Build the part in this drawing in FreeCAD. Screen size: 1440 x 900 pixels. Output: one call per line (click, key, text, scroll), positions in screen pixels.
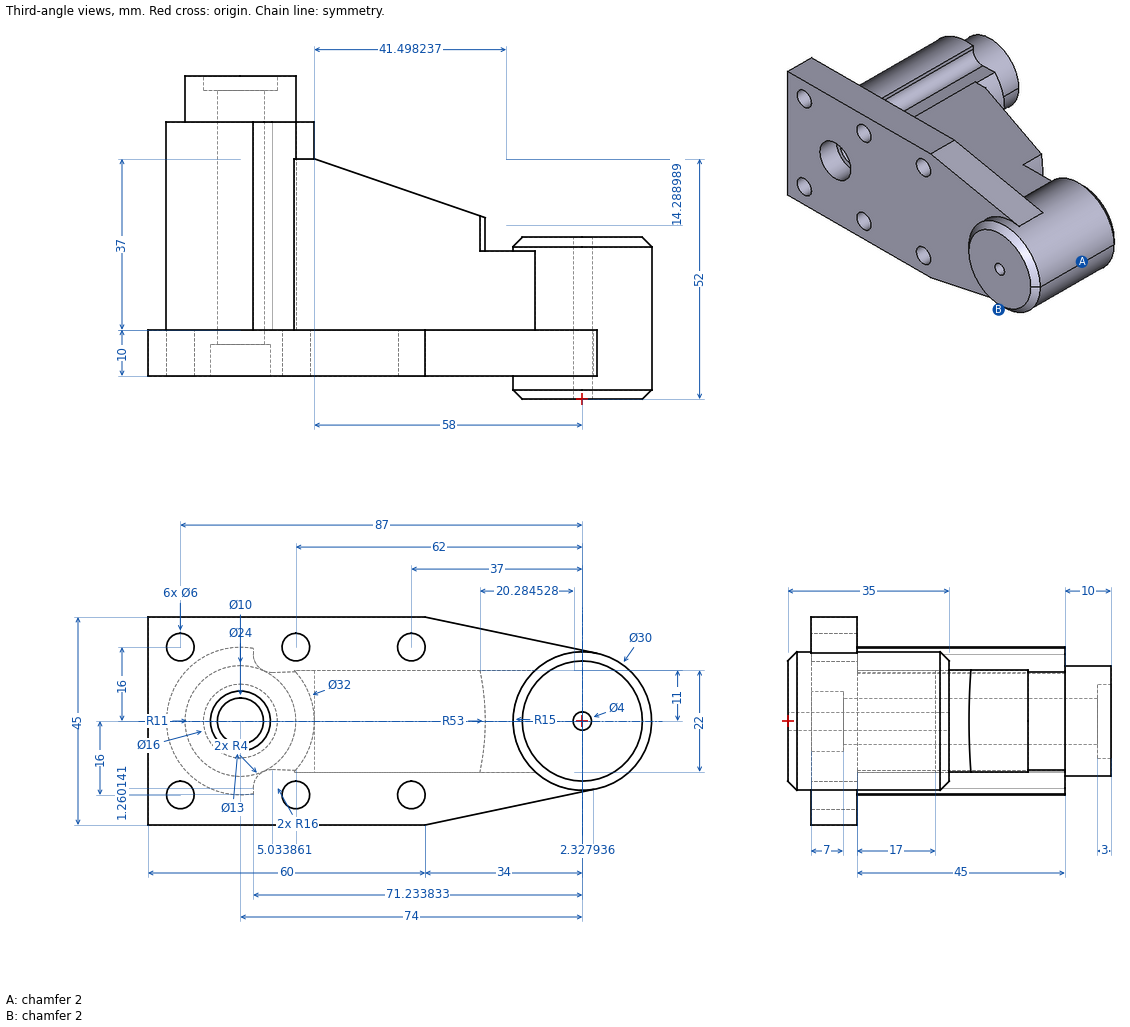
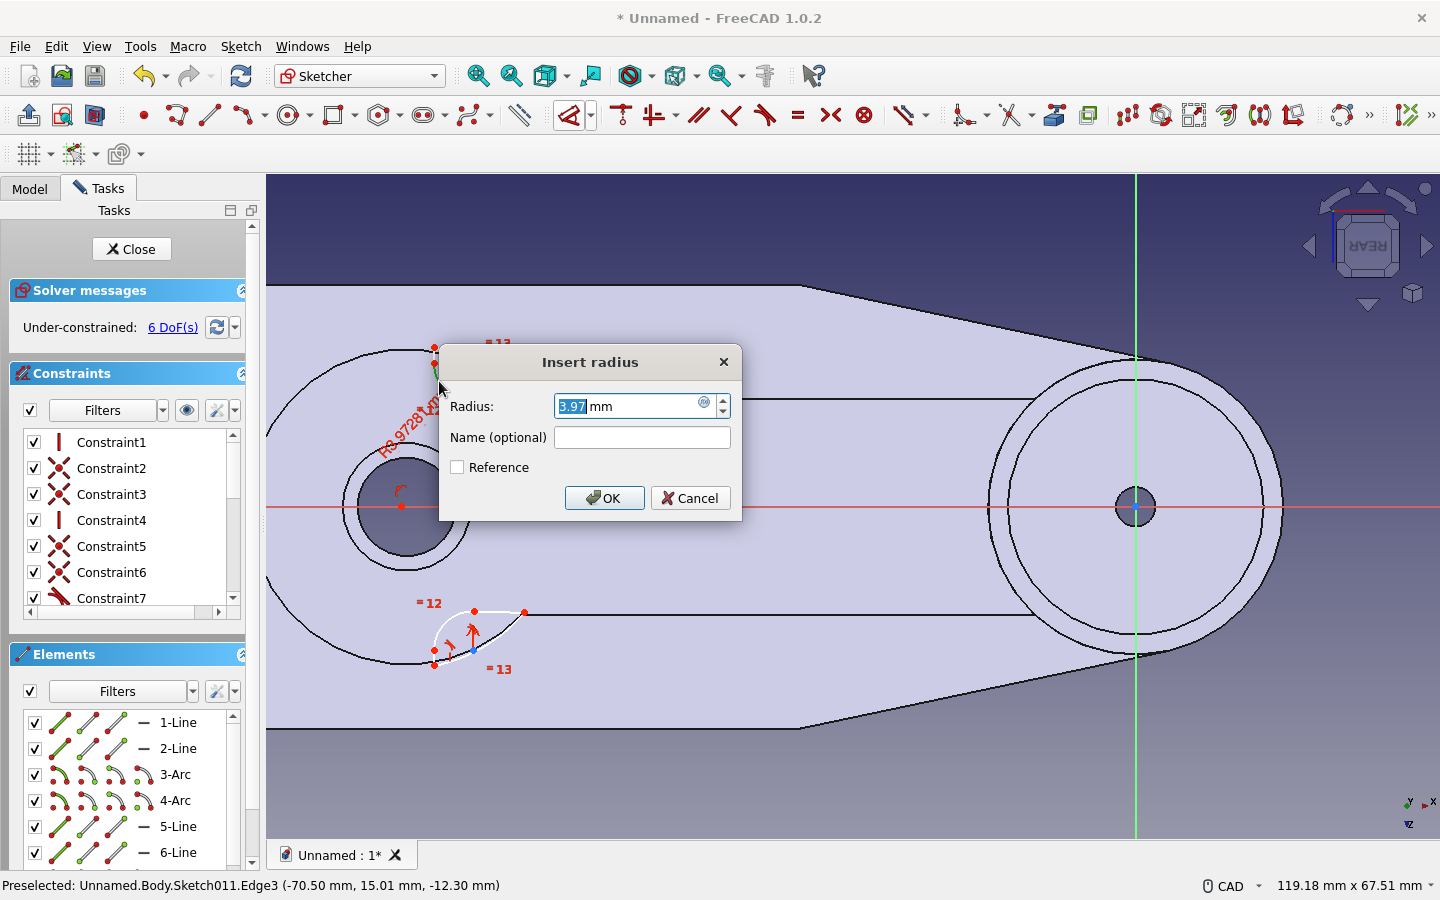
text(4)
key(Return)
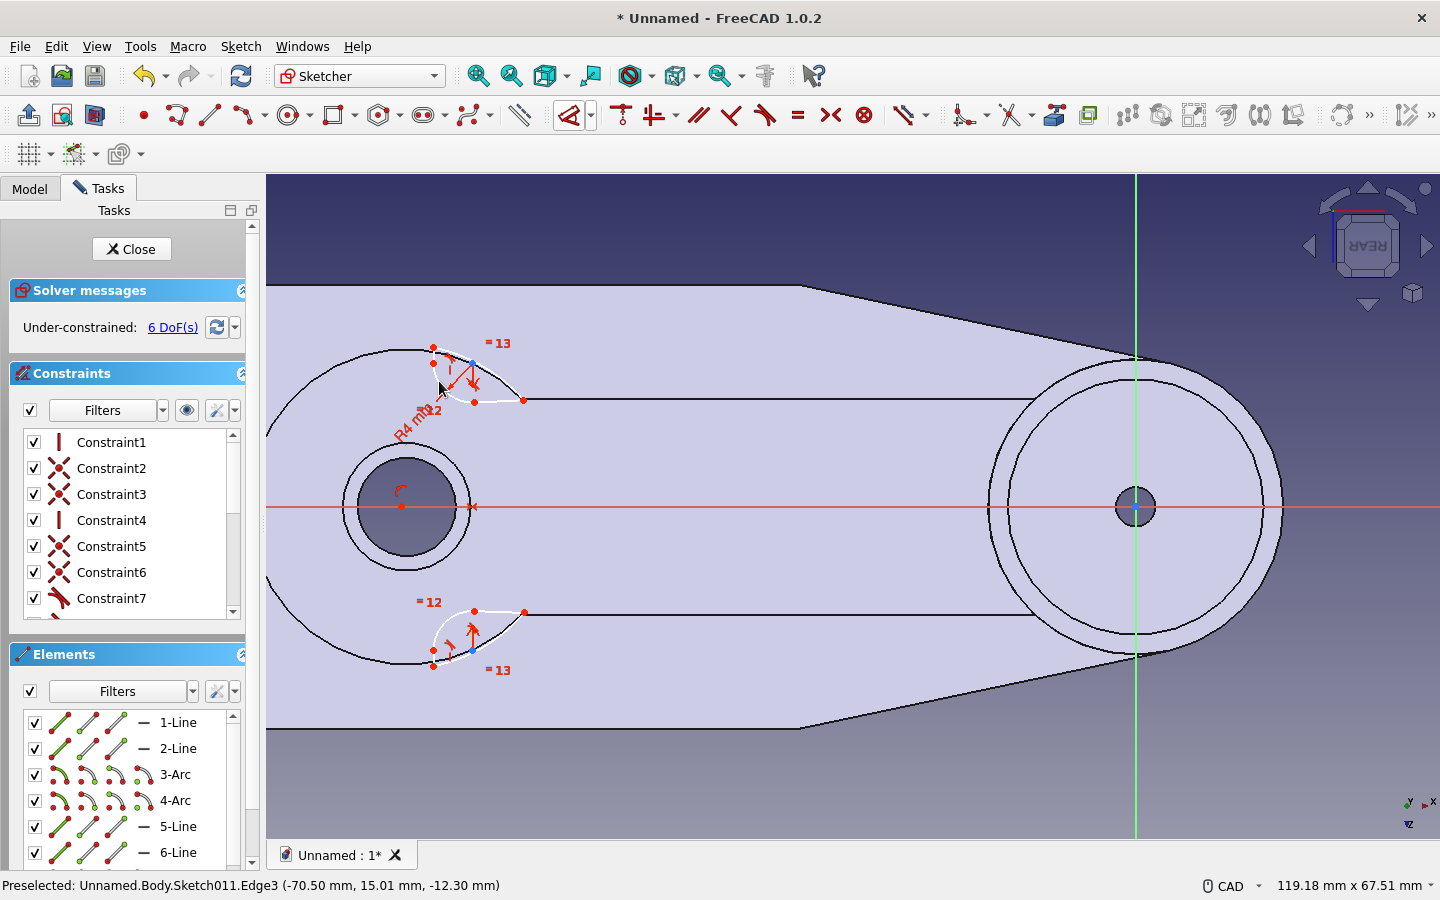
click(501, 378)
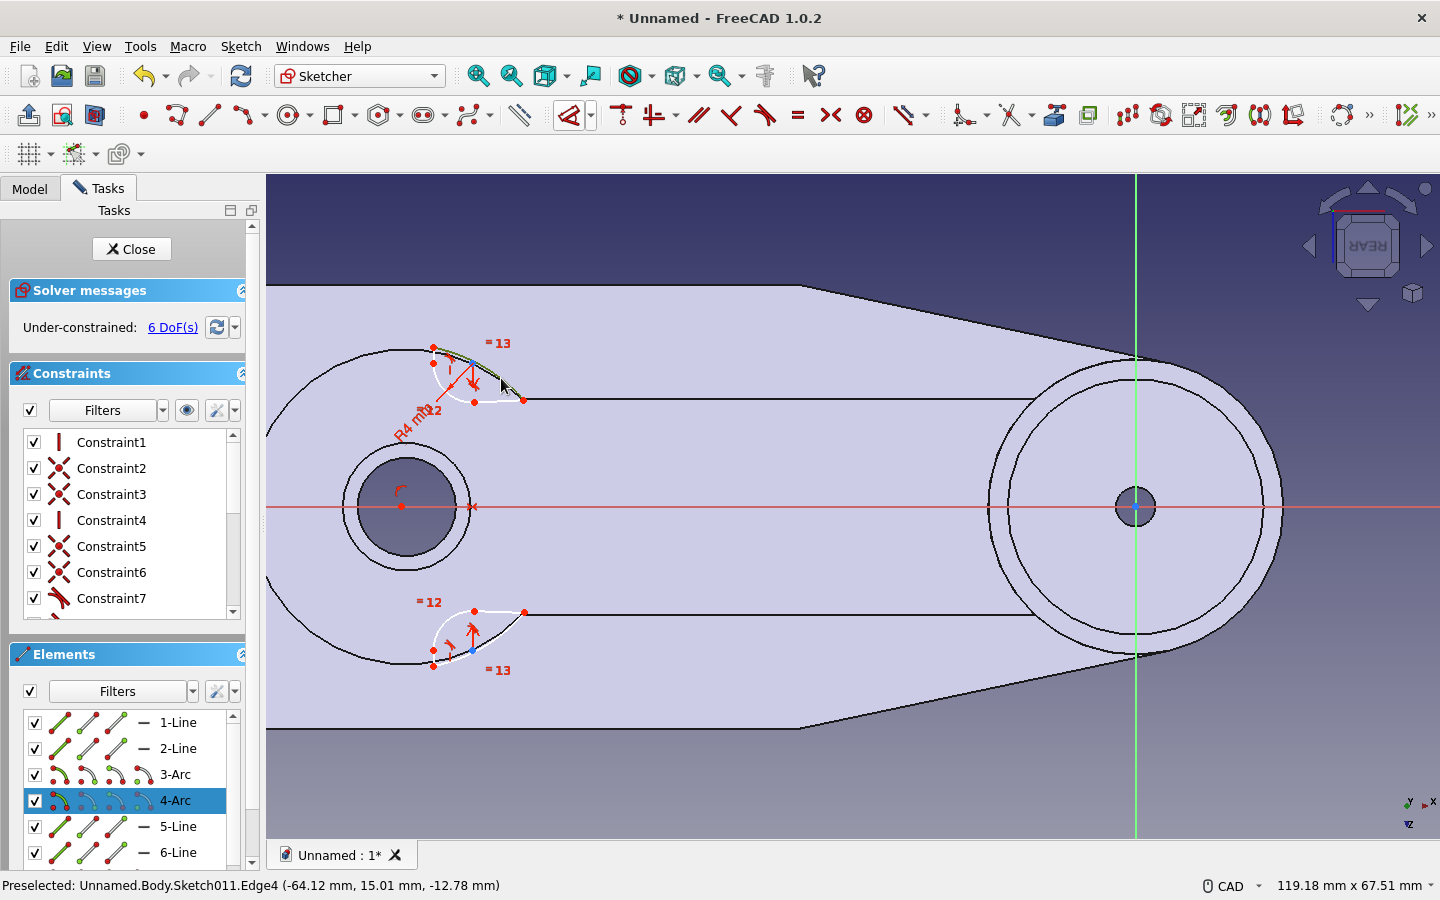
click(590, 116)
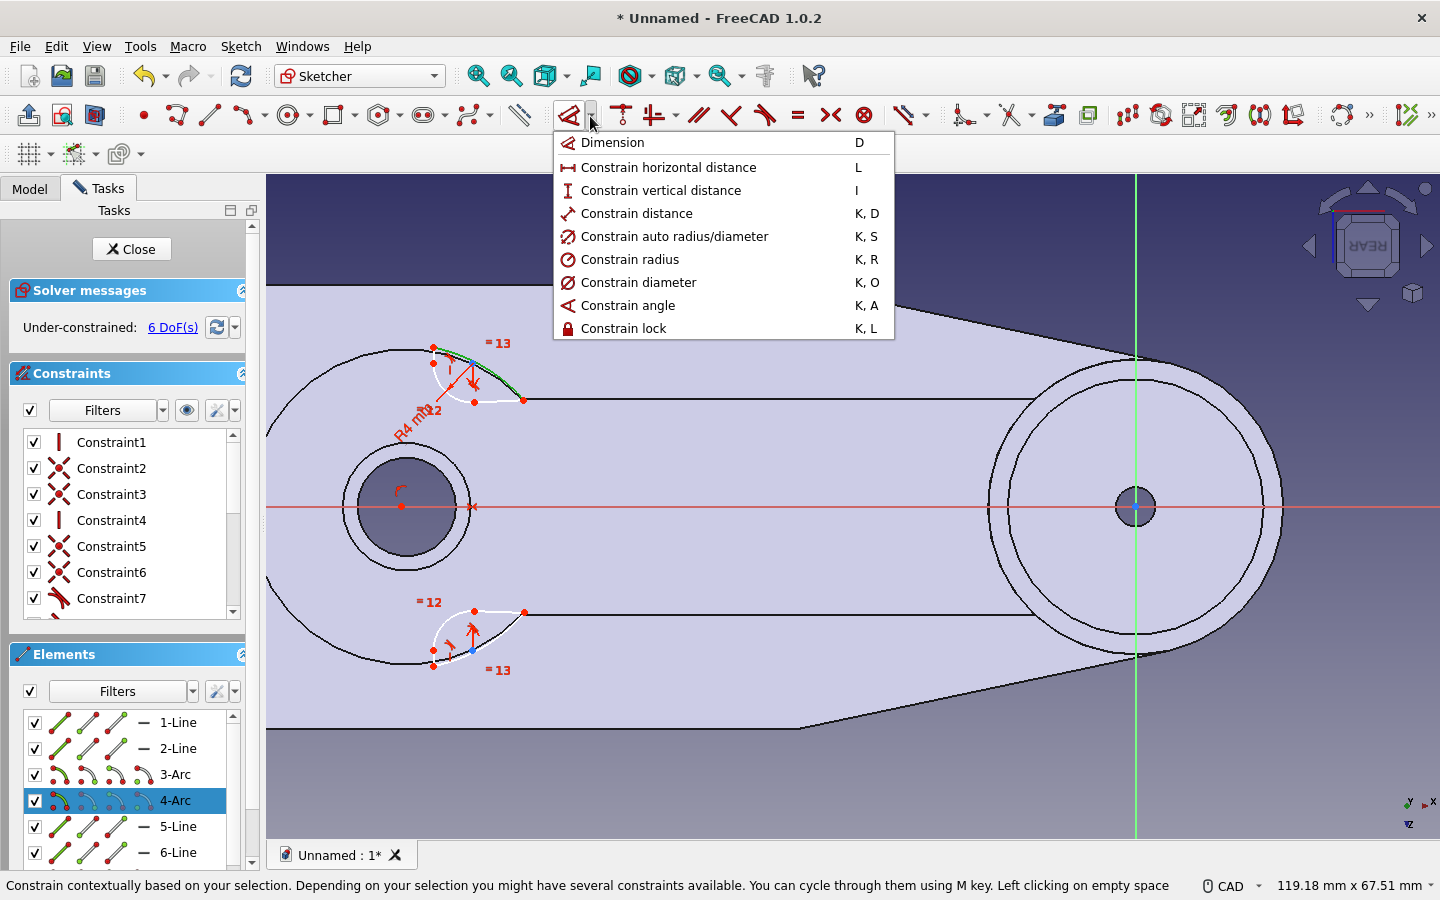
click(724, 260)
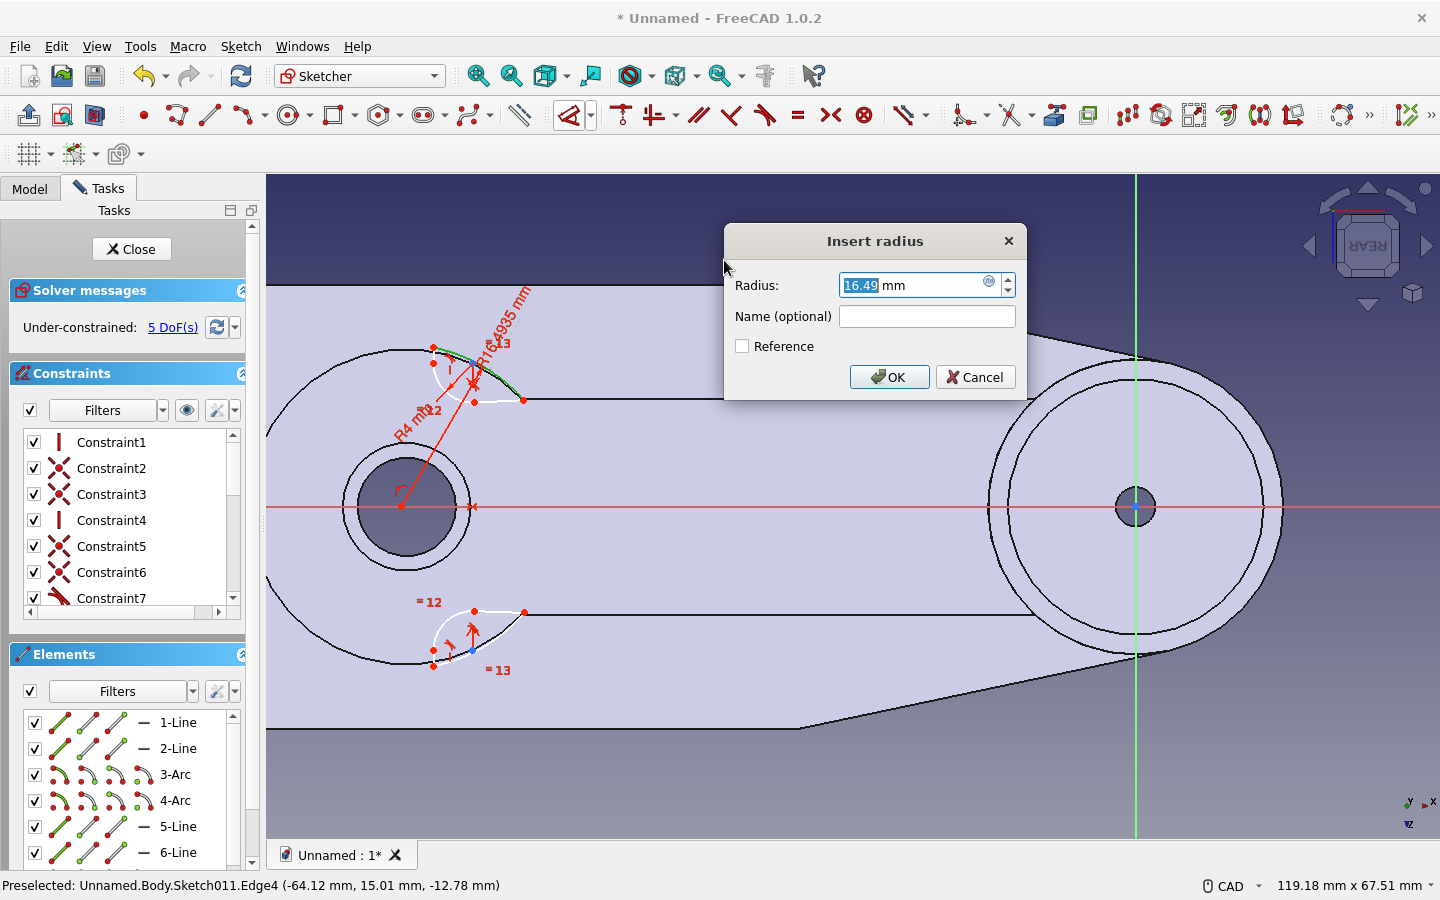
text(16)
key(Return)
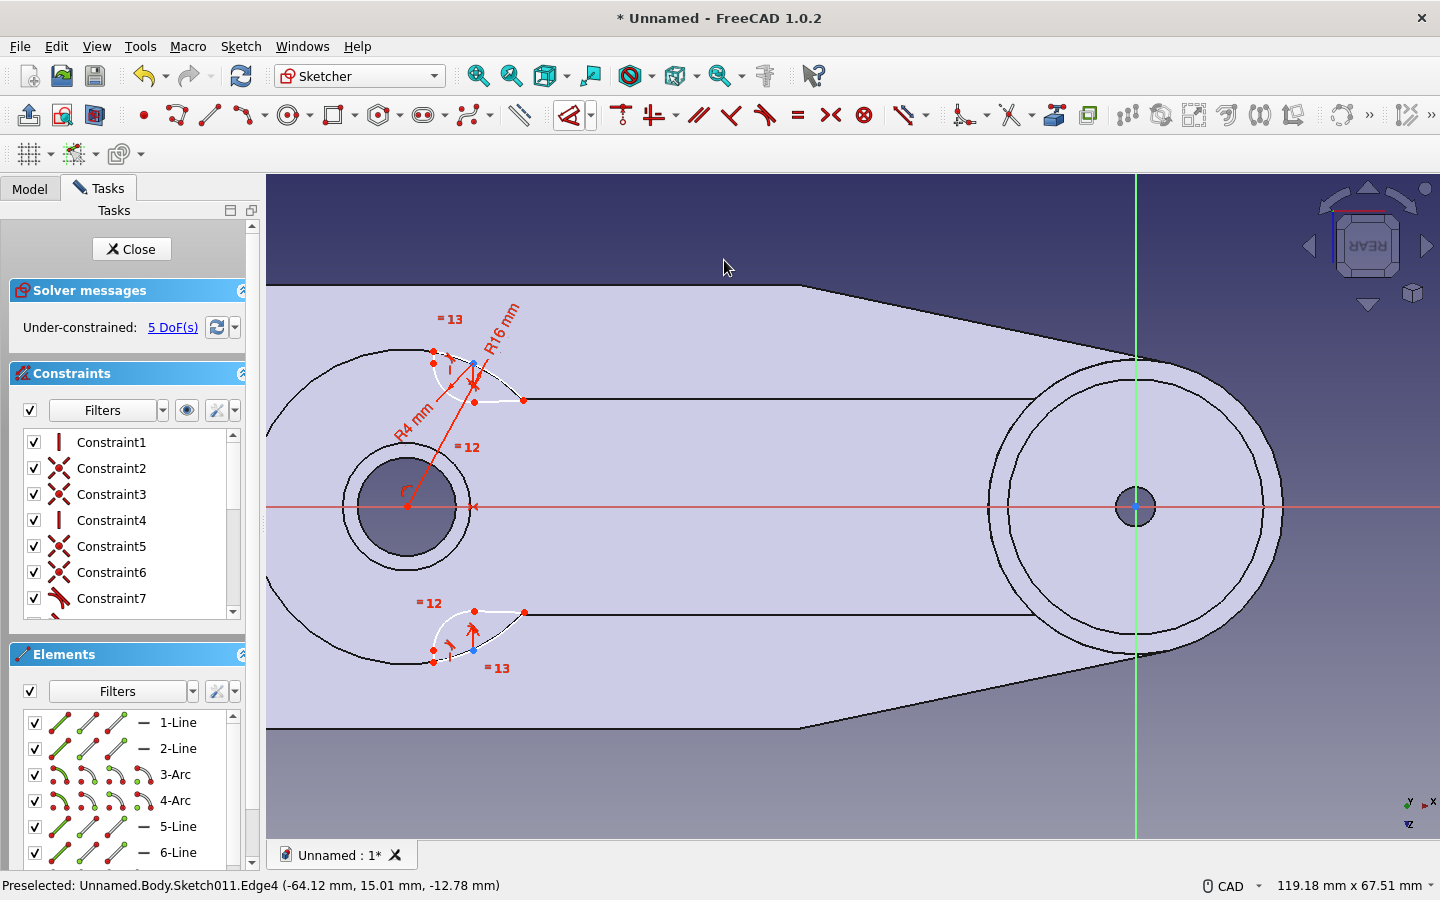
click(407, 507)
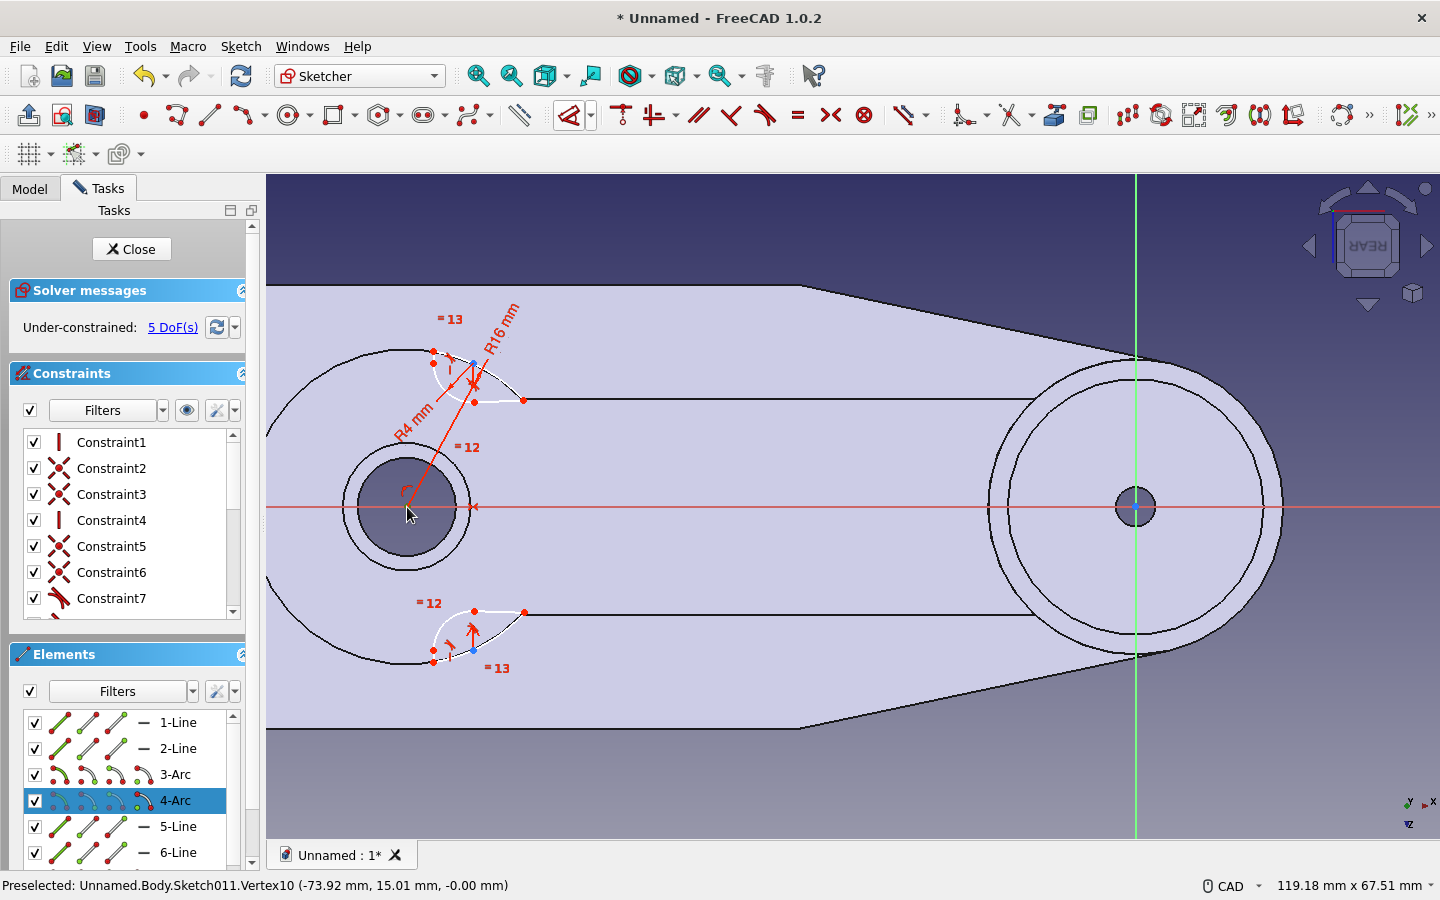
click(590, 116)